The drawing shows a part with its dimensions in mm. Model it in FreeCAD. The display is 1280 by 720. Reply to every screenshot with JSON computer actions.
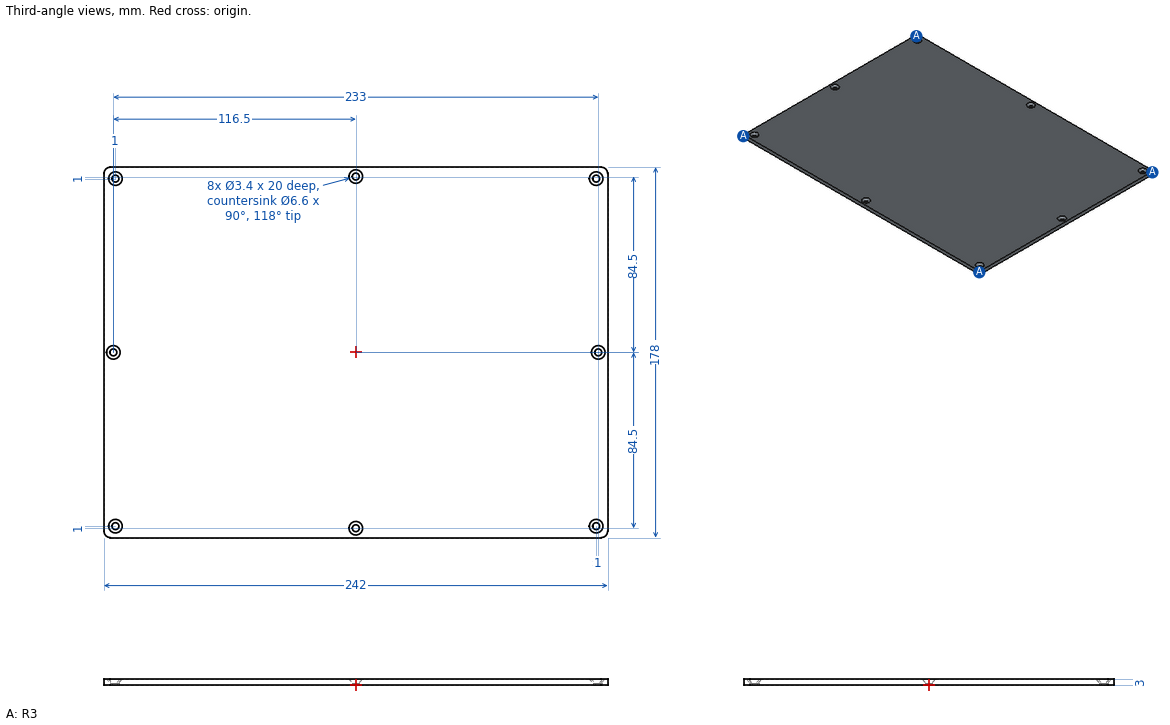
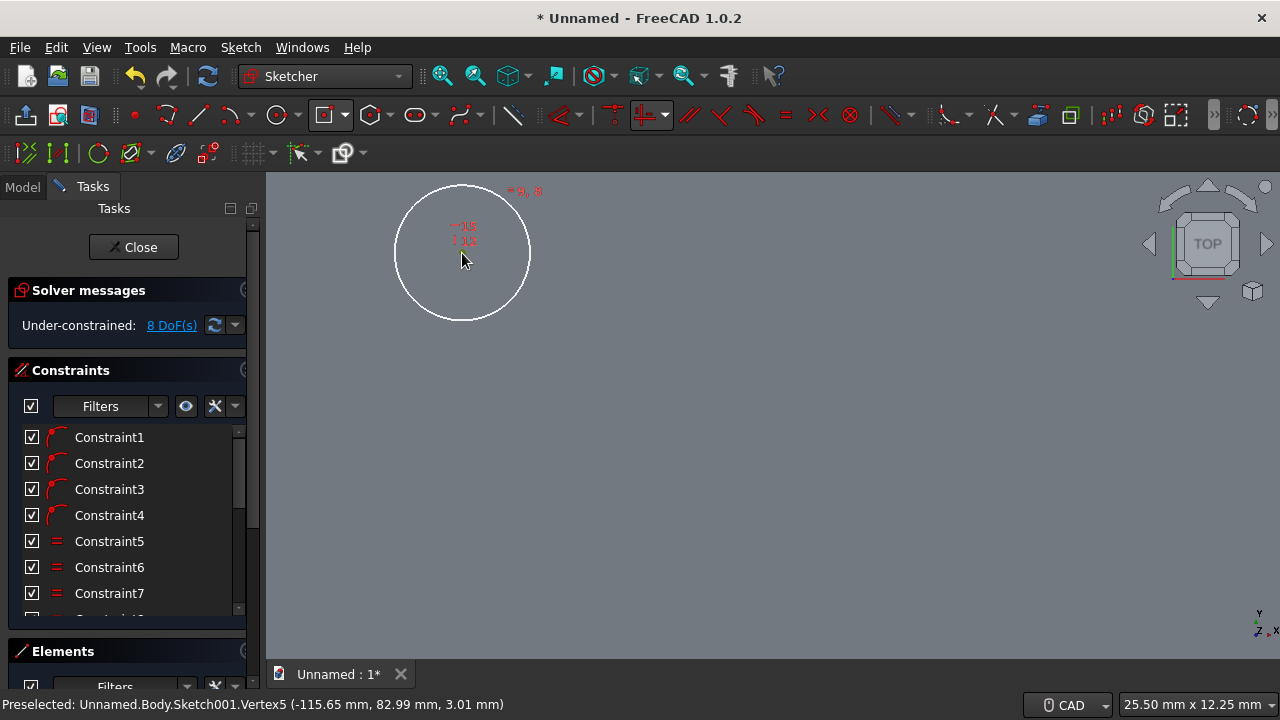
{"action": "key", "text": "l"}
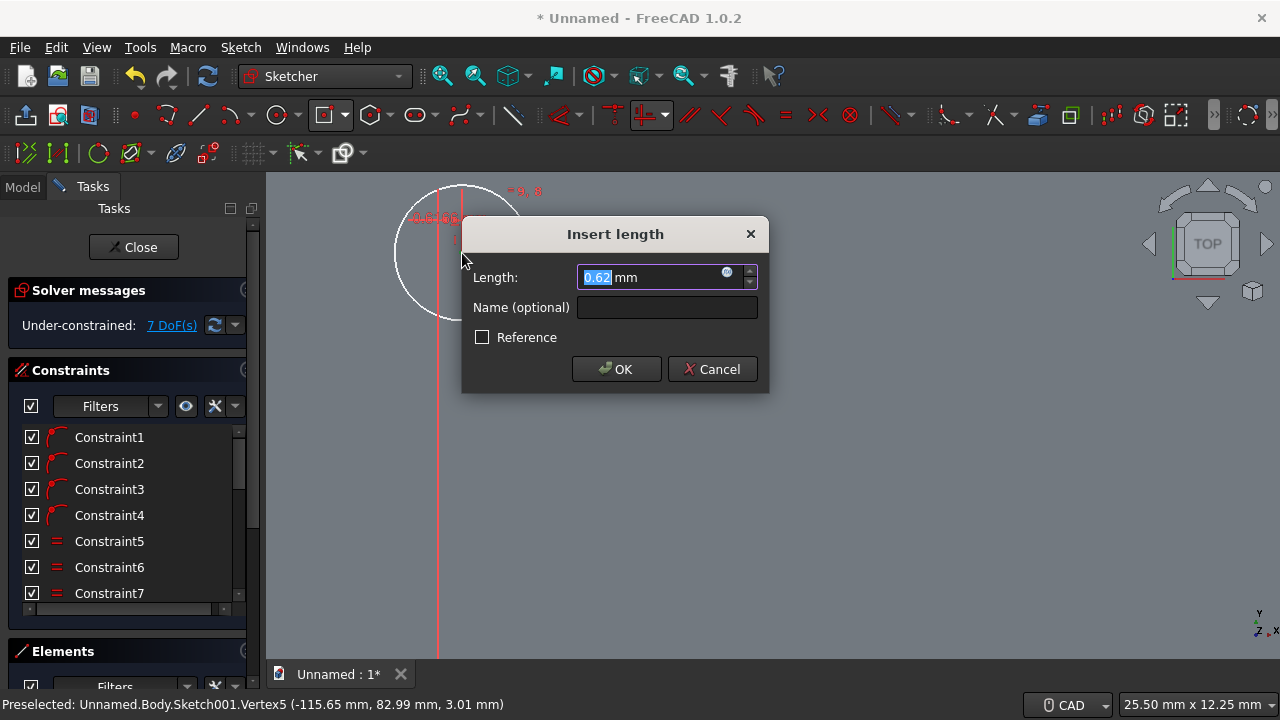
{"action": "type", "text": "1"}
{"action": "key", "text": "Return"}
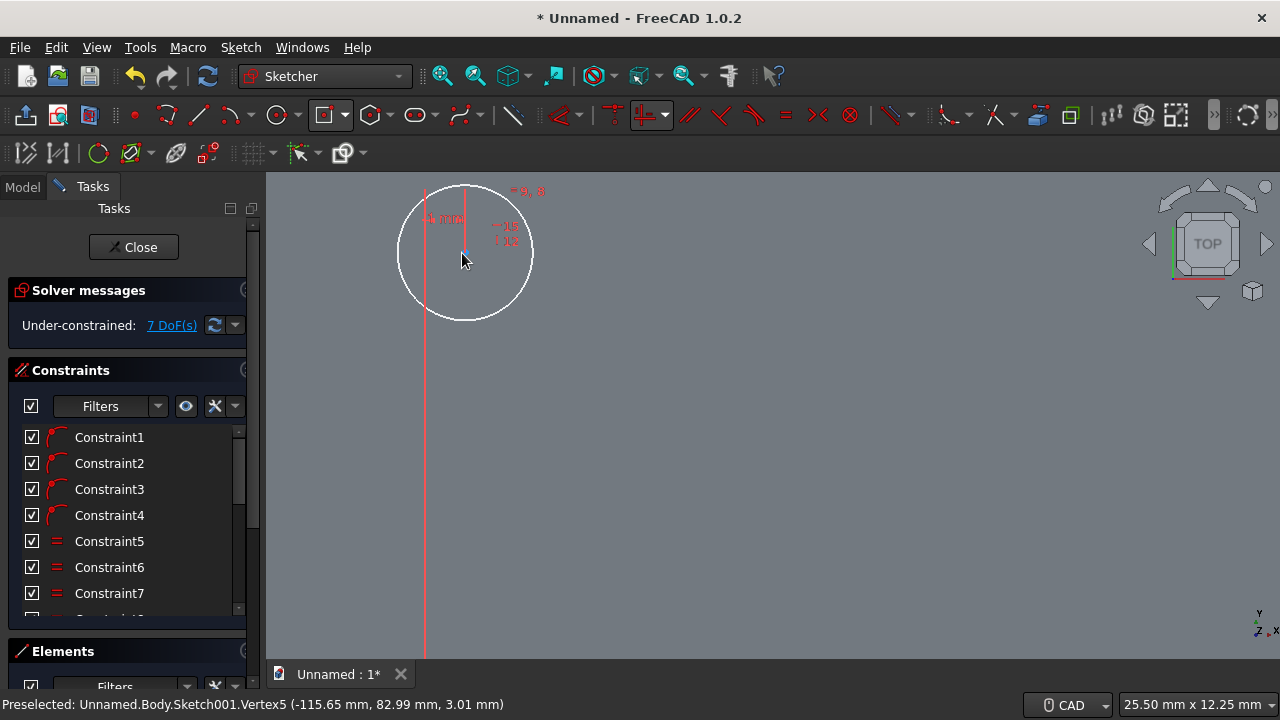
{"action": "scroll", "coordinate": [476, 251], "scroll_direction": "down", "scroll_amount": 15}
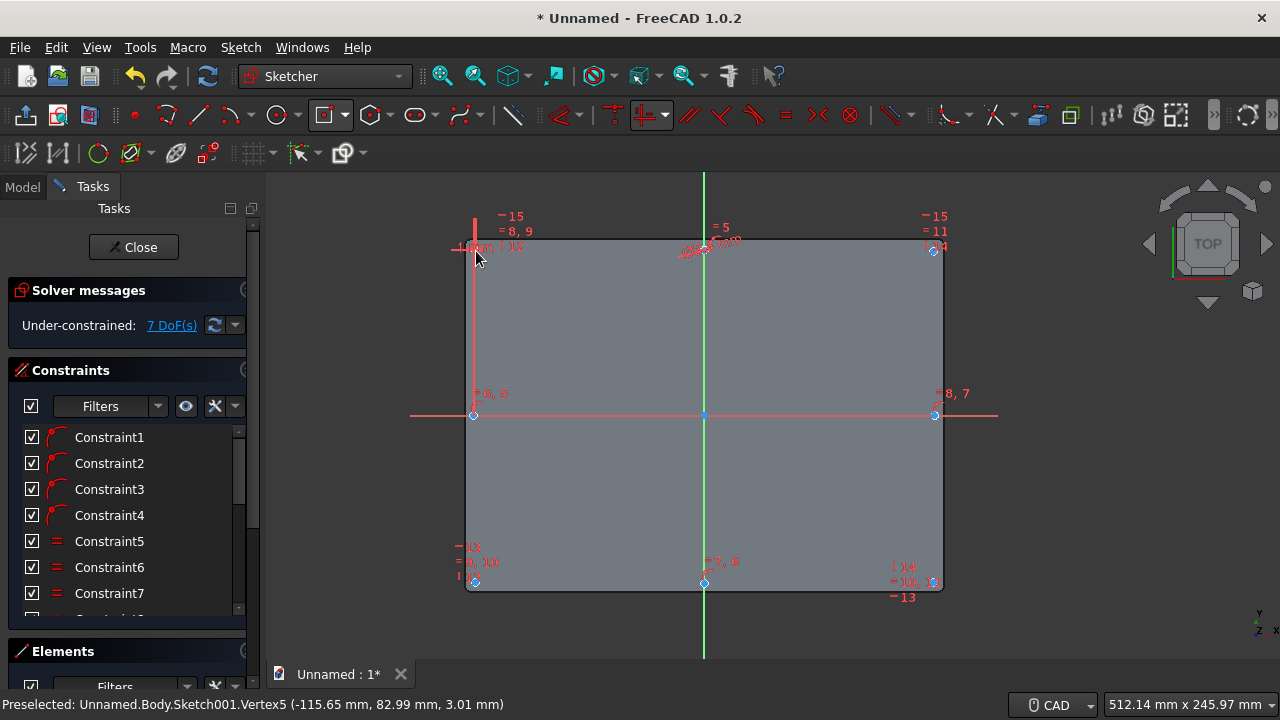
{"action": "scroll", "coordinate": [704, 250], "scroll_direction": "up", "scroll_amount": 15}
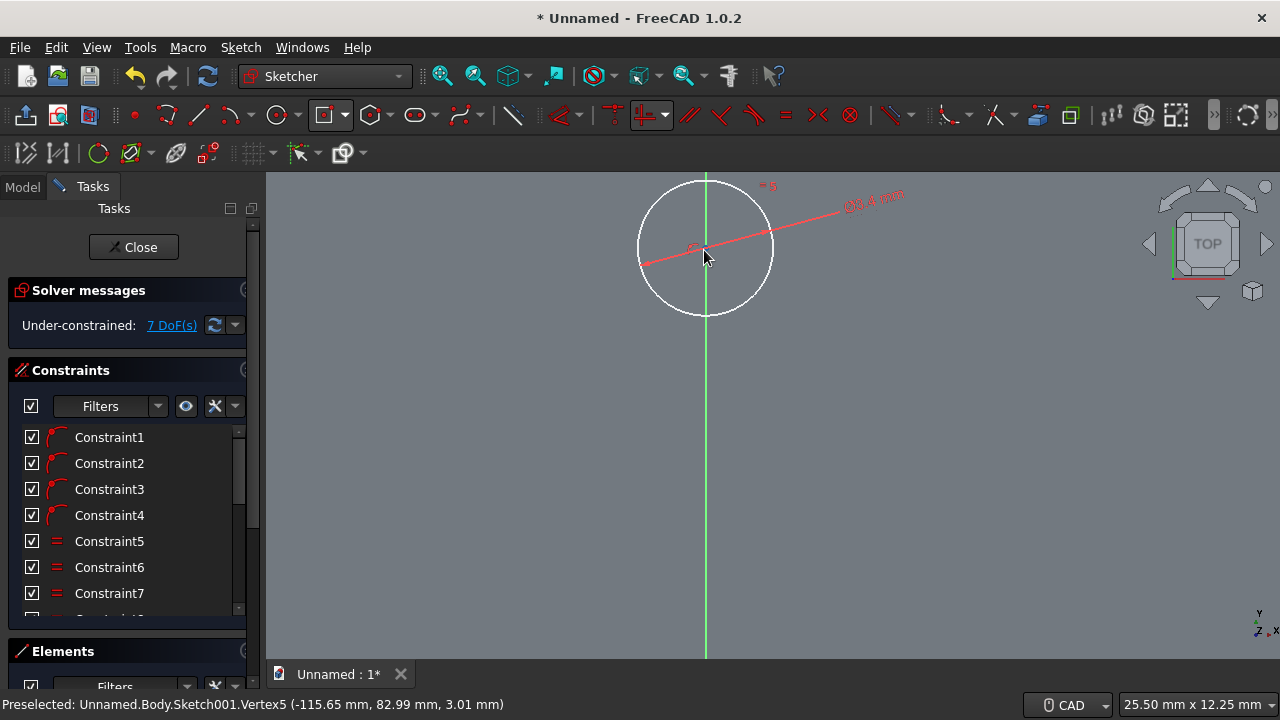
{"action": "left_click", "coordinate": [706, 248]}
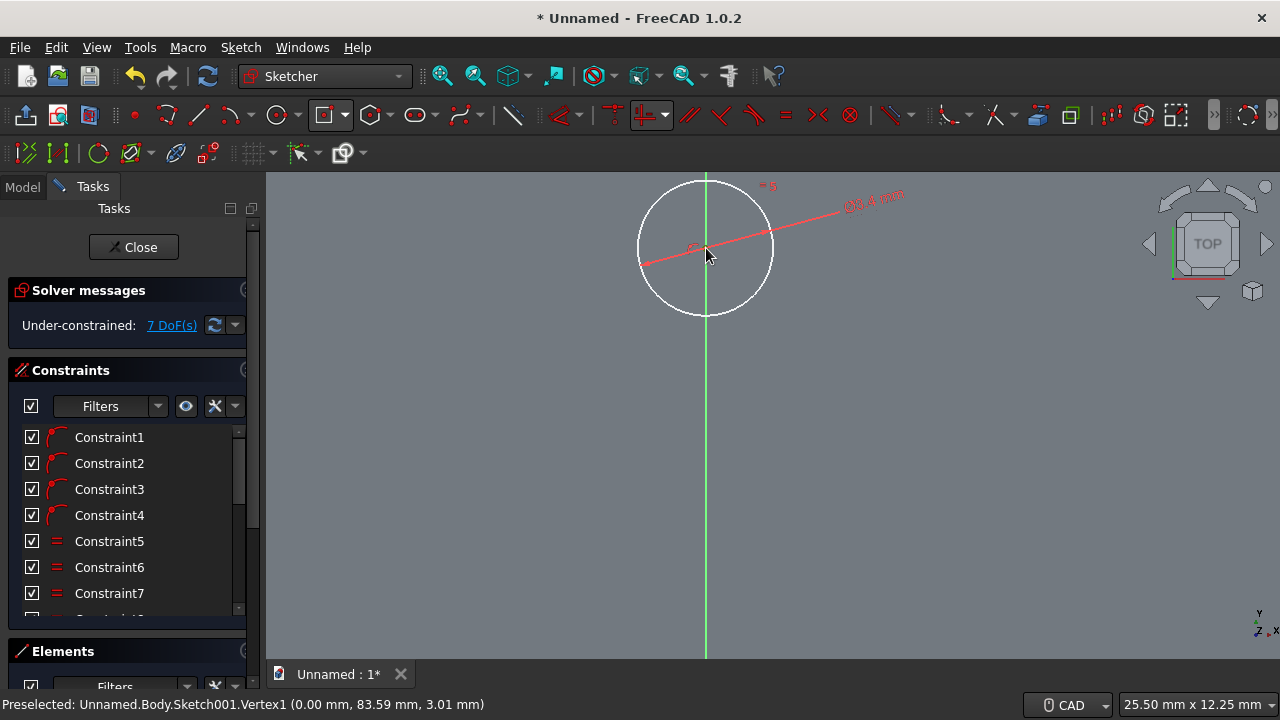
{"action": "scroll", "coordinate": [704, 250], "scroll_direction": "down", "scroll_amount": 15}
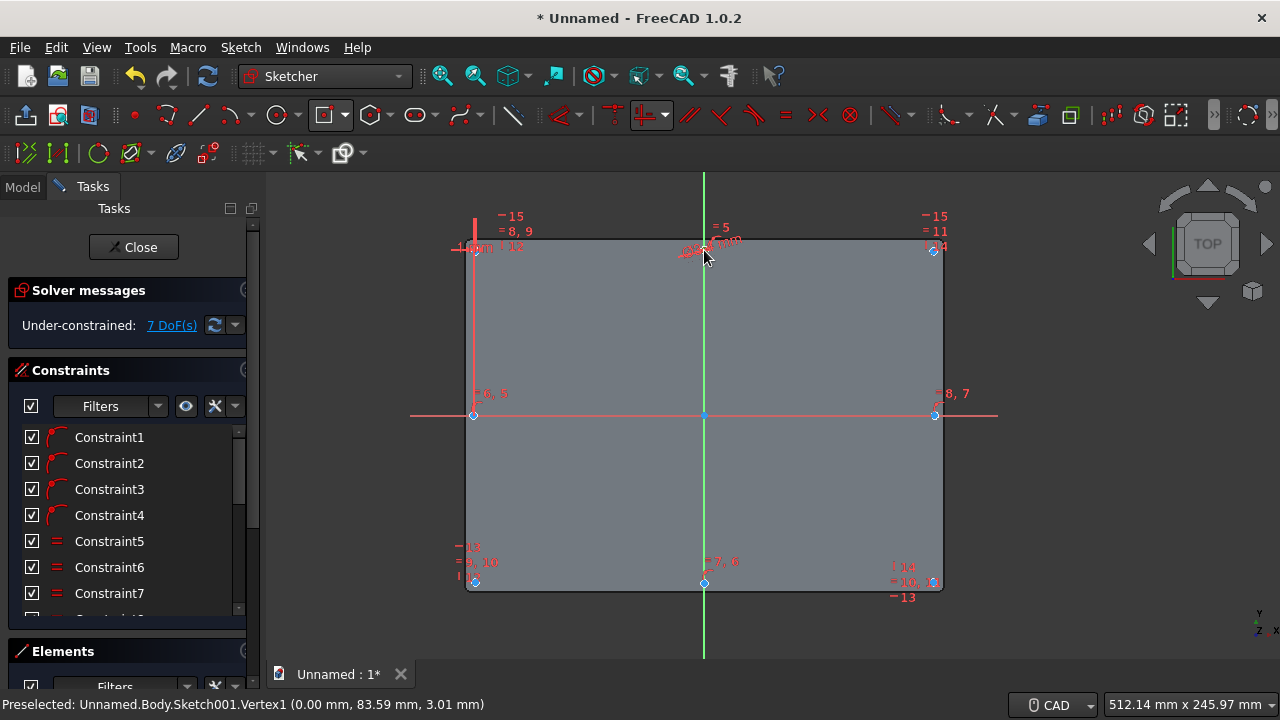
{"action": "scroll", "coordinate": [476, 251], "scroll_direction": "up", "scroll_amount": 15}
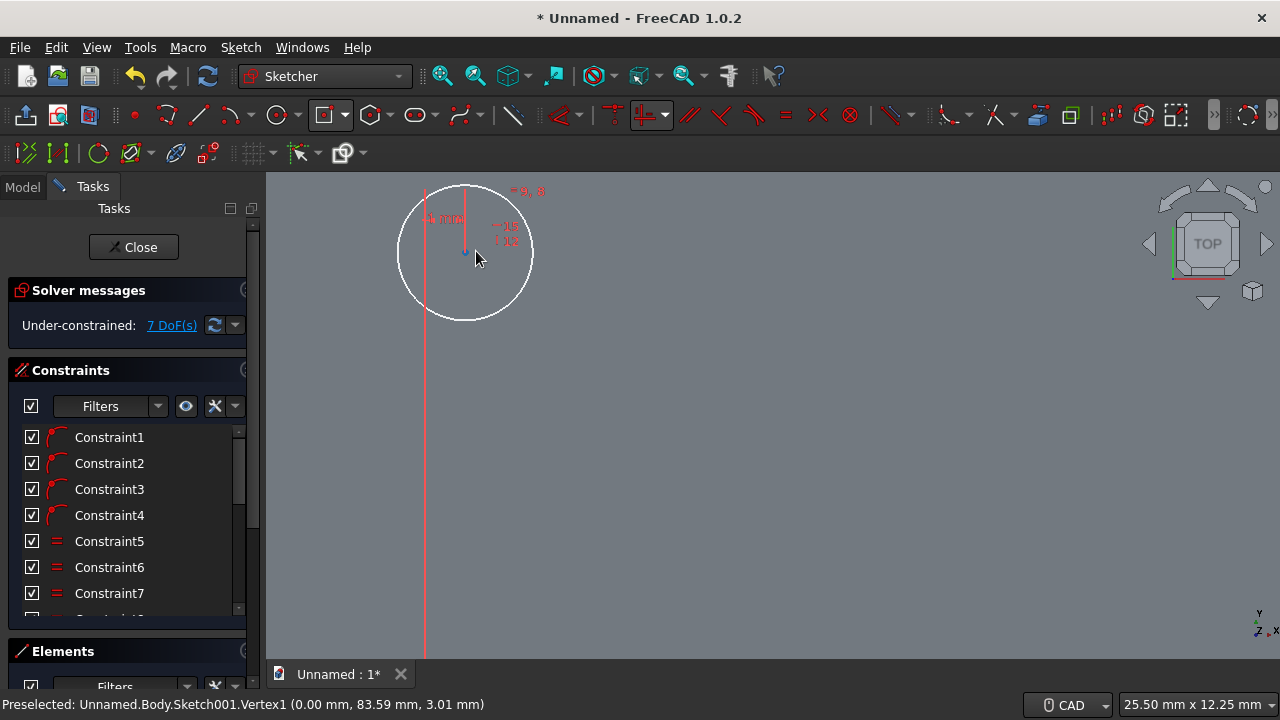
{"action": "left_click", "coordinate": [465, 253]}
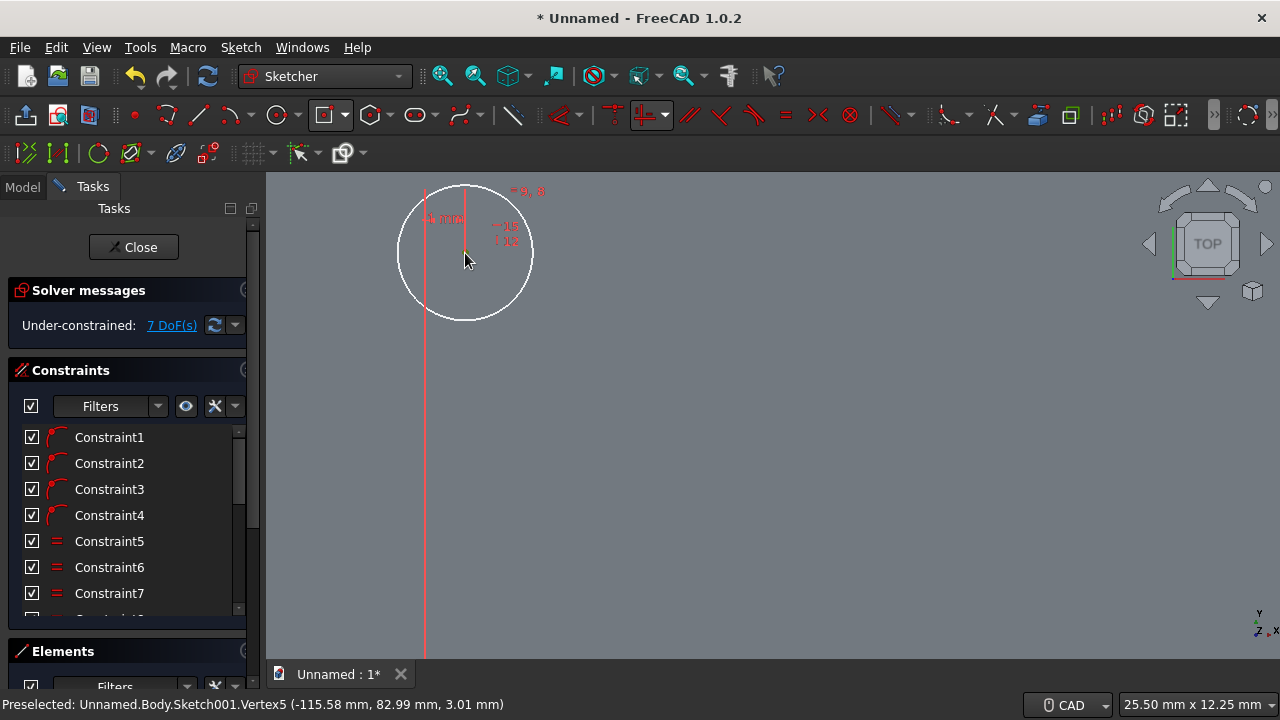
{"action": "key", "text": "i"}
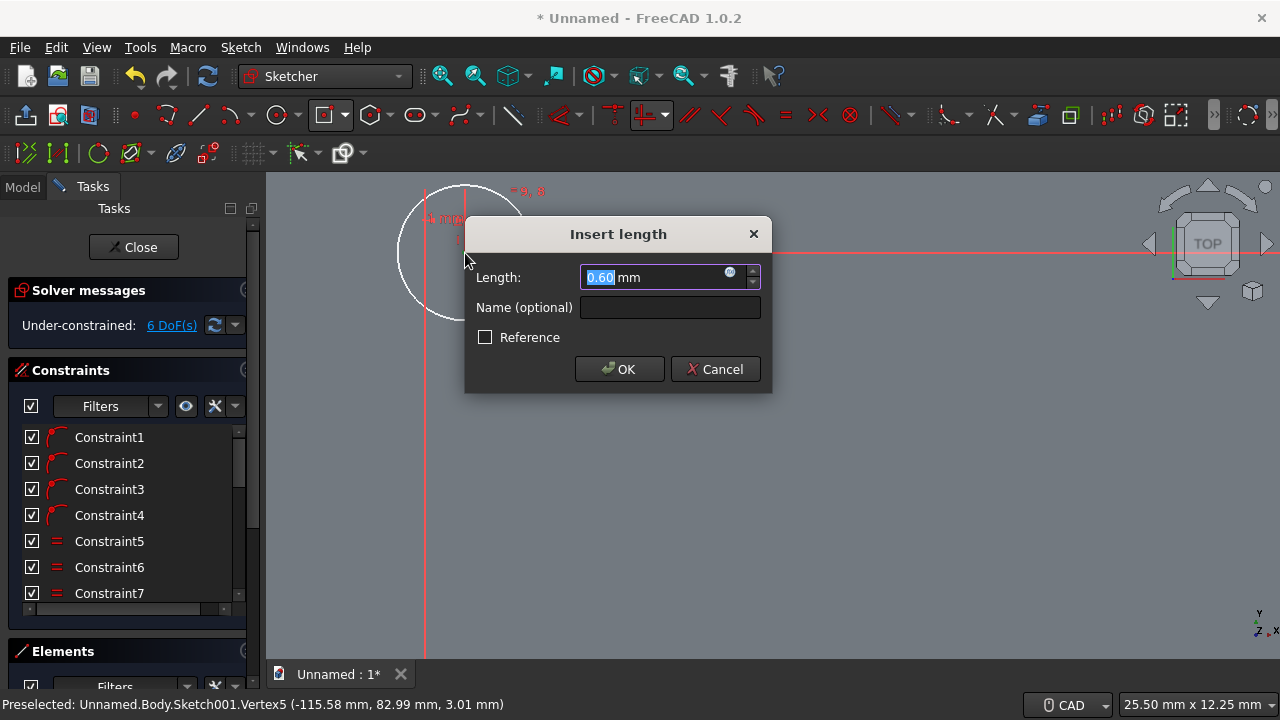
{"action": "type", "text": "1"}
{"action": "key", "text": "Return"}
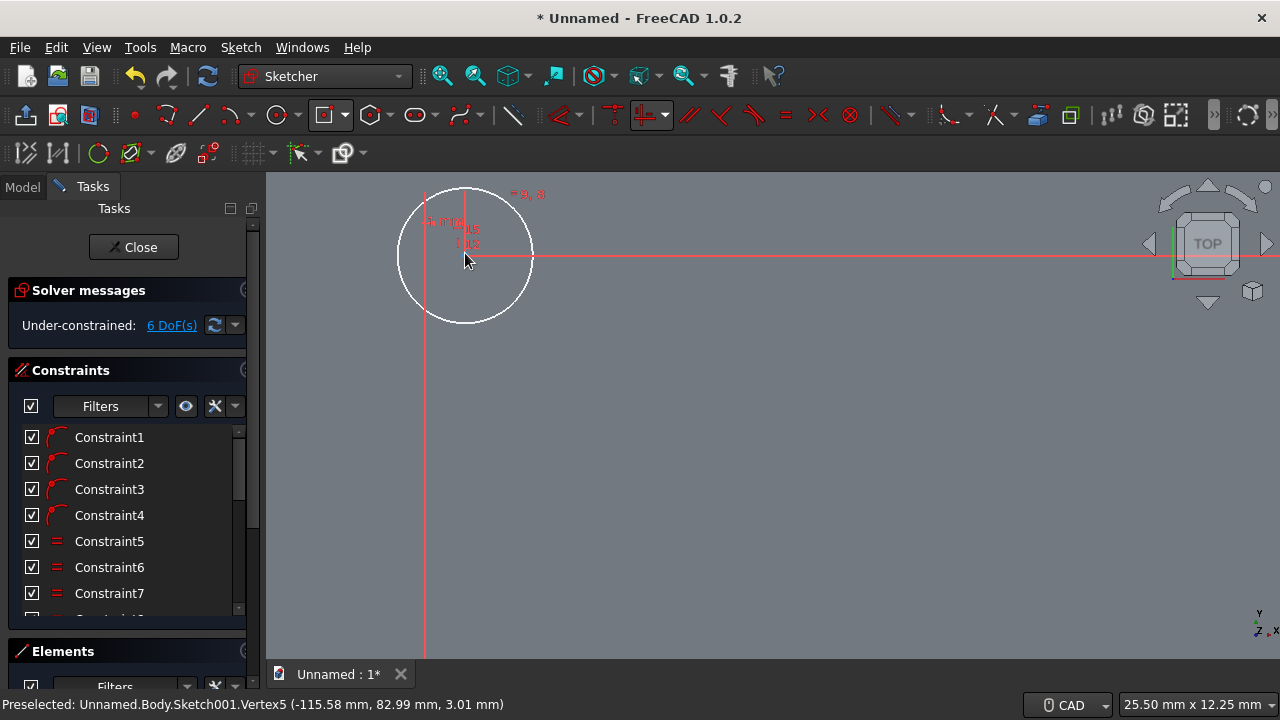
{"action": "scroll", "coordinate": [476, 251], "scroll_direction": "down", "scroll_amount": 15}